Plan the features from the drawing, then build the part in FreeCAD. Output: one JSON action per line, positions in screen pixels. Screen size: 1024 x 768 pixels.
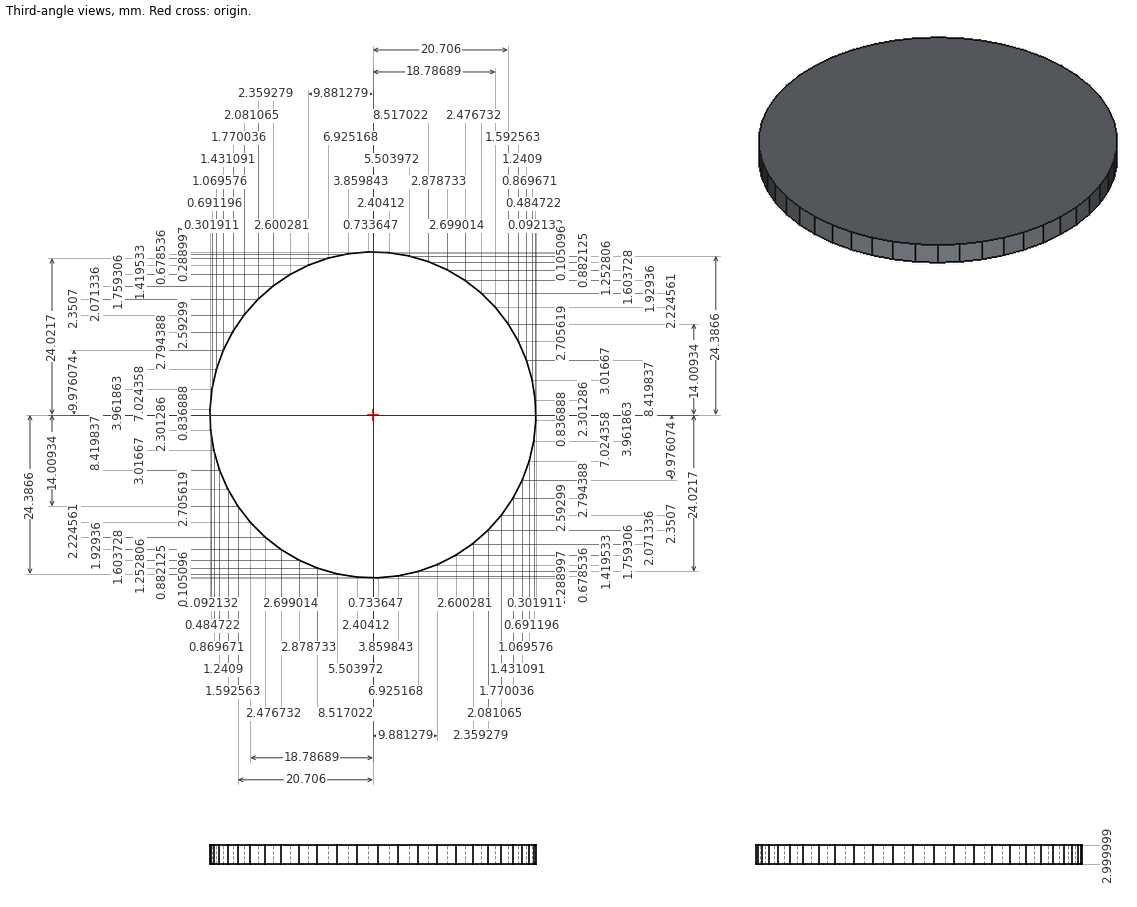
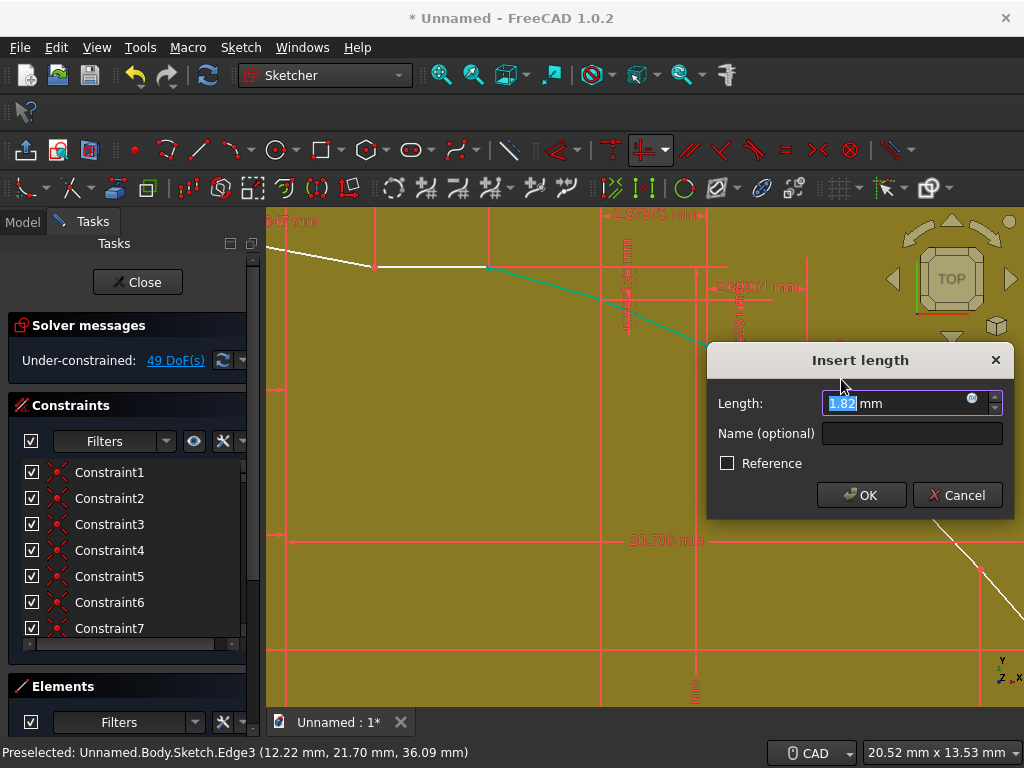
{"action": "type", "text": "1.603728"}
{"action": "key", "text": "Return"}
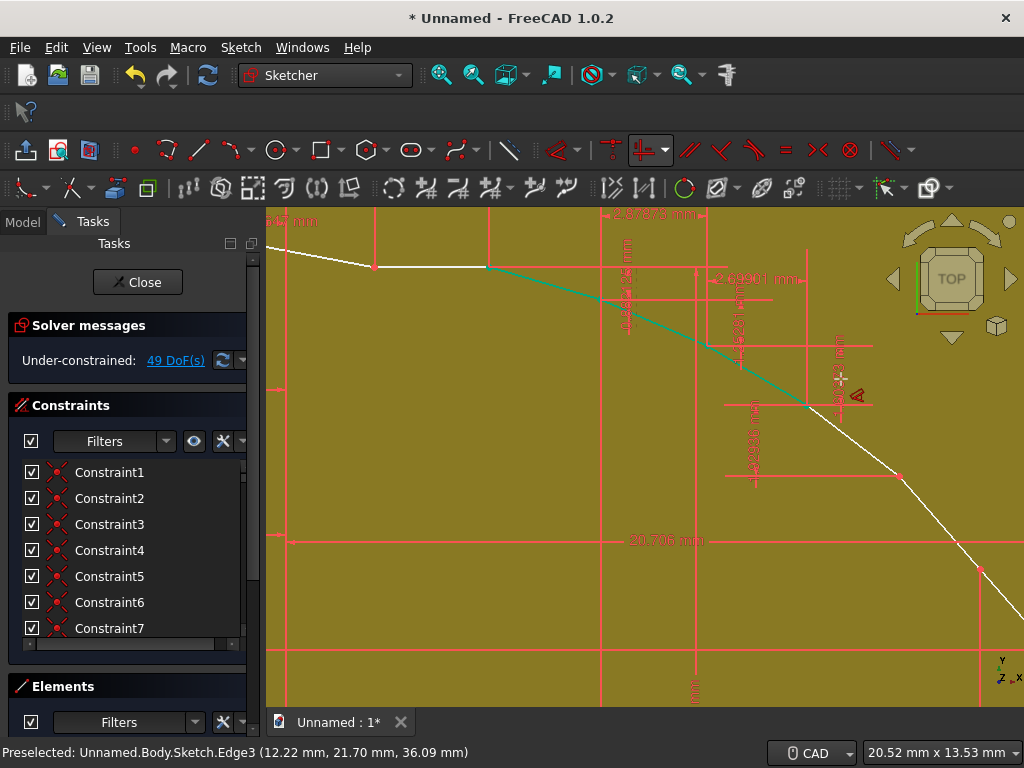
{"action": "left_click", "coordinate": [835, 427]}
{"action": "left_click", "coordinate": [833, 510]}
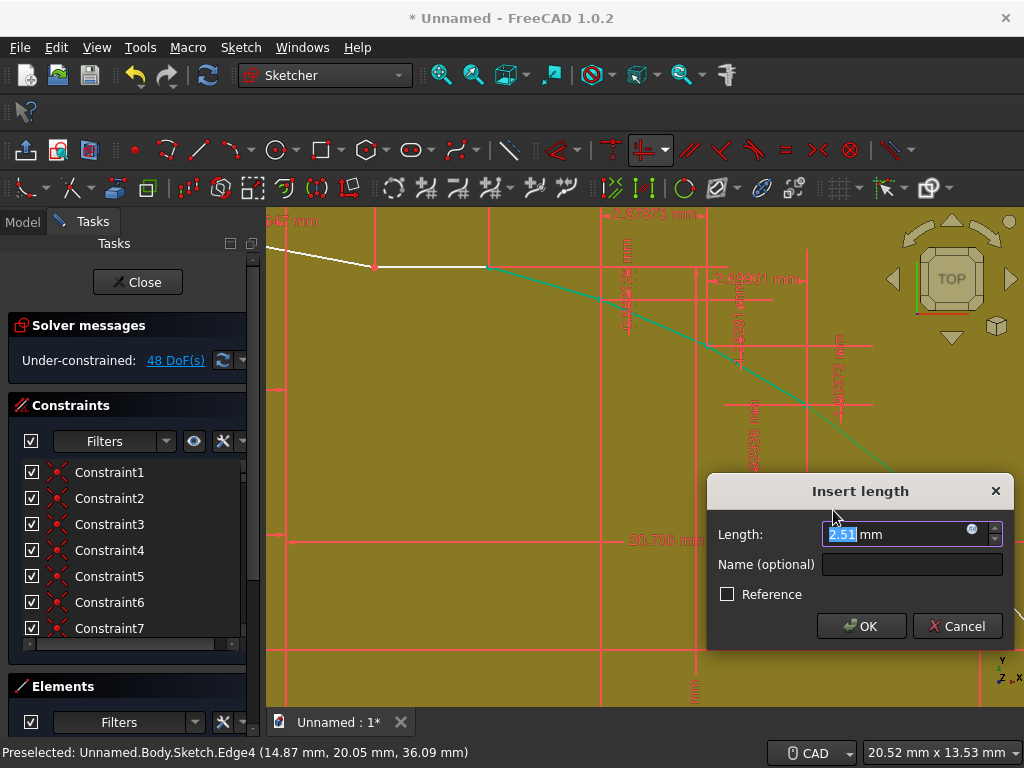
{"action": "type", "text": "2.476732"}
{"action": "key", "text": "Return"}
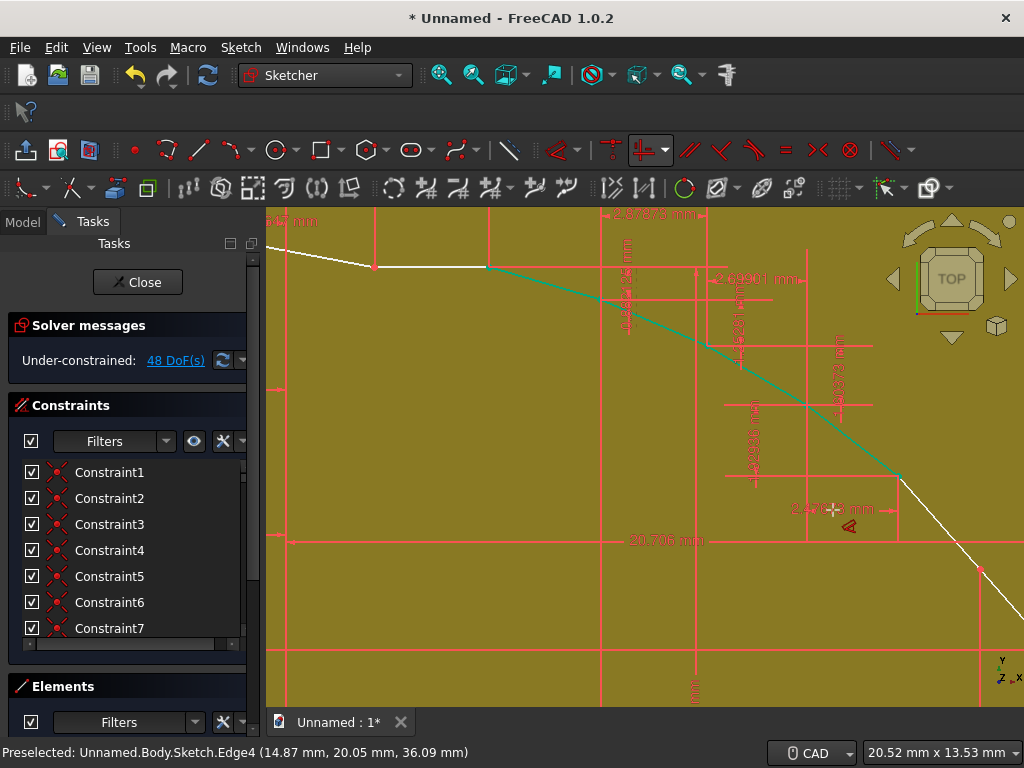
{"action": "scroll", "coordinate": [634, 316], "scroll_direction": "down", "scroll_amount": 9}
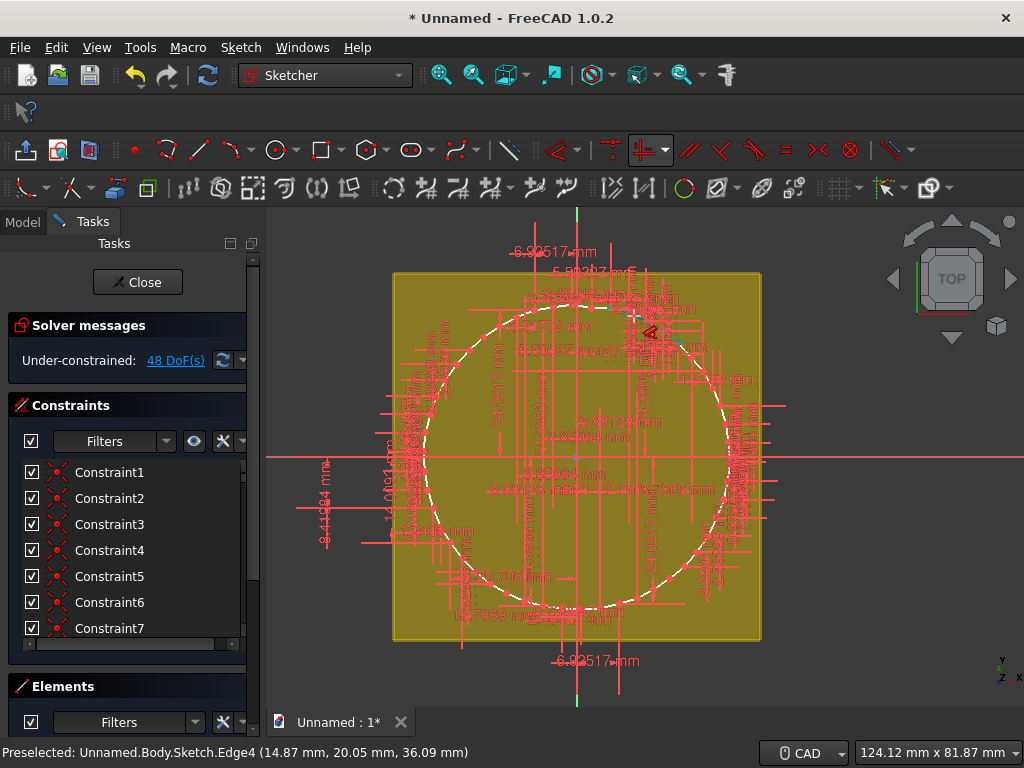
{"action": "scroll", "coordinate": [682, 347], "scroll_direction": "up", "scroll_amount": 6}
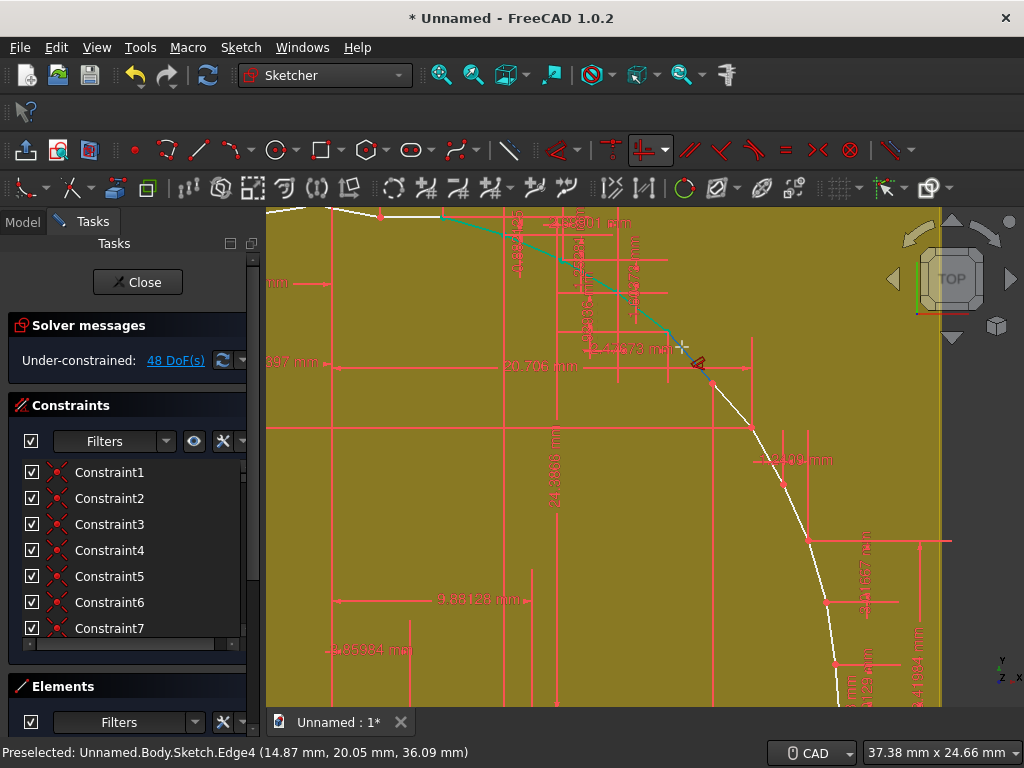
{"action": "left_click", "coordinate": [681, 347]}
{"action": "left_click", "coordinate": [747, 358]}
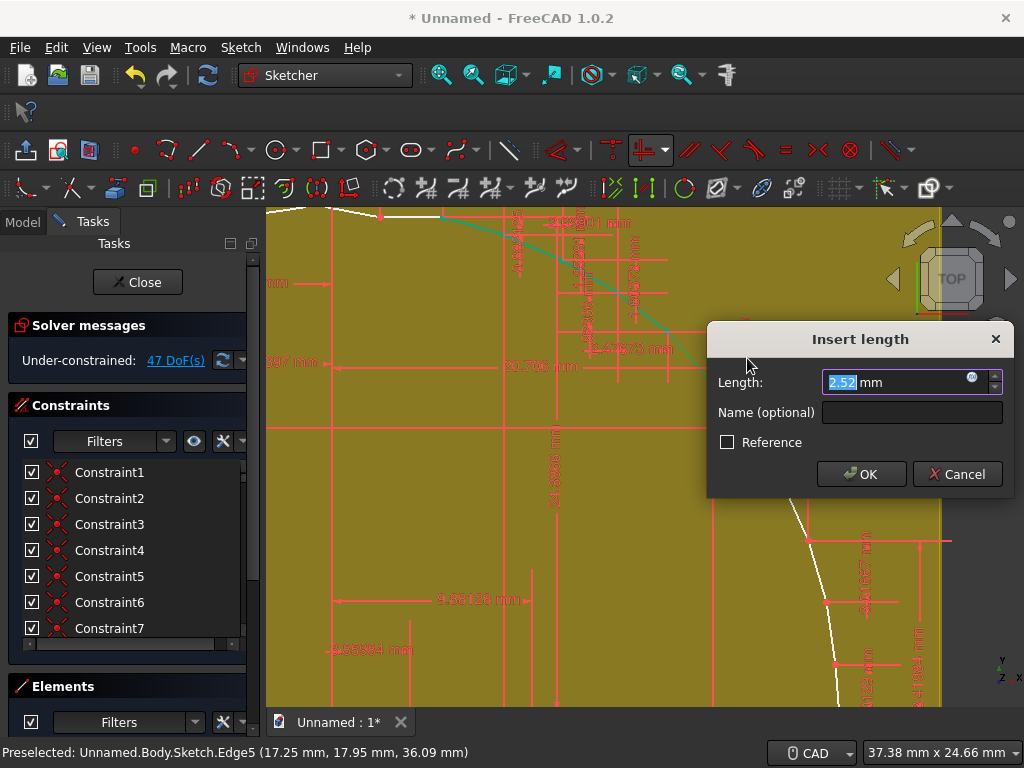
{"action": "type", "text": "2.224561"}
{"action": "key", "text": "Return"}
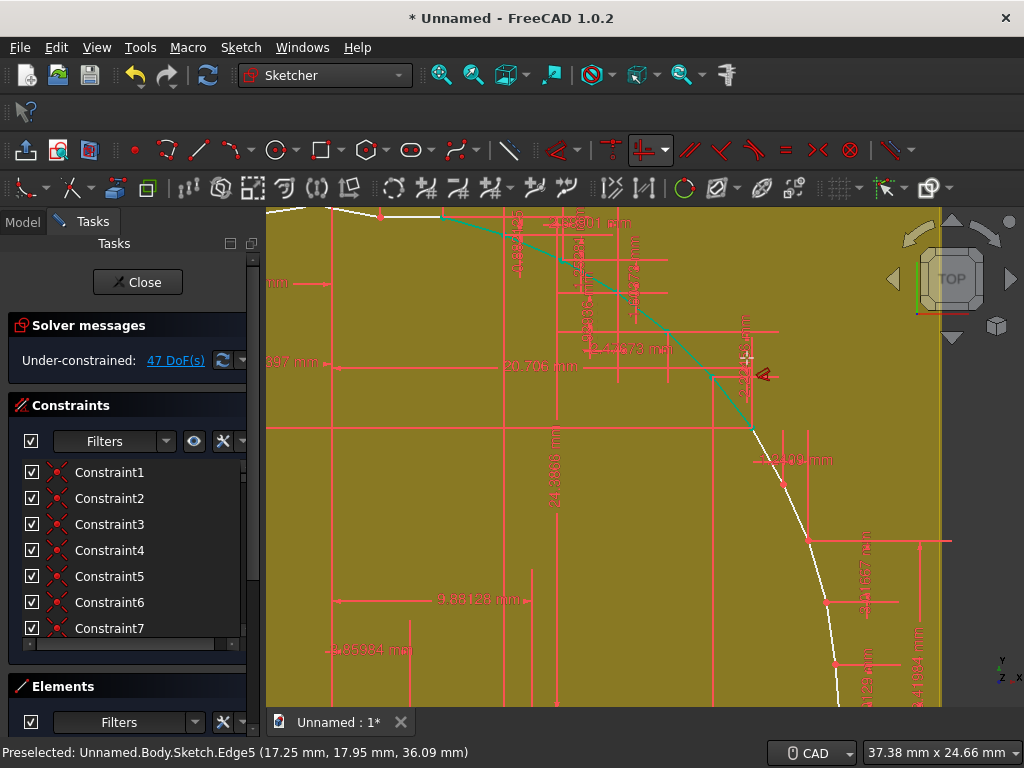
{"action": "scroll", "coordinate": [761, 445], "scroll_direction": "up", "scroll_amount": 2}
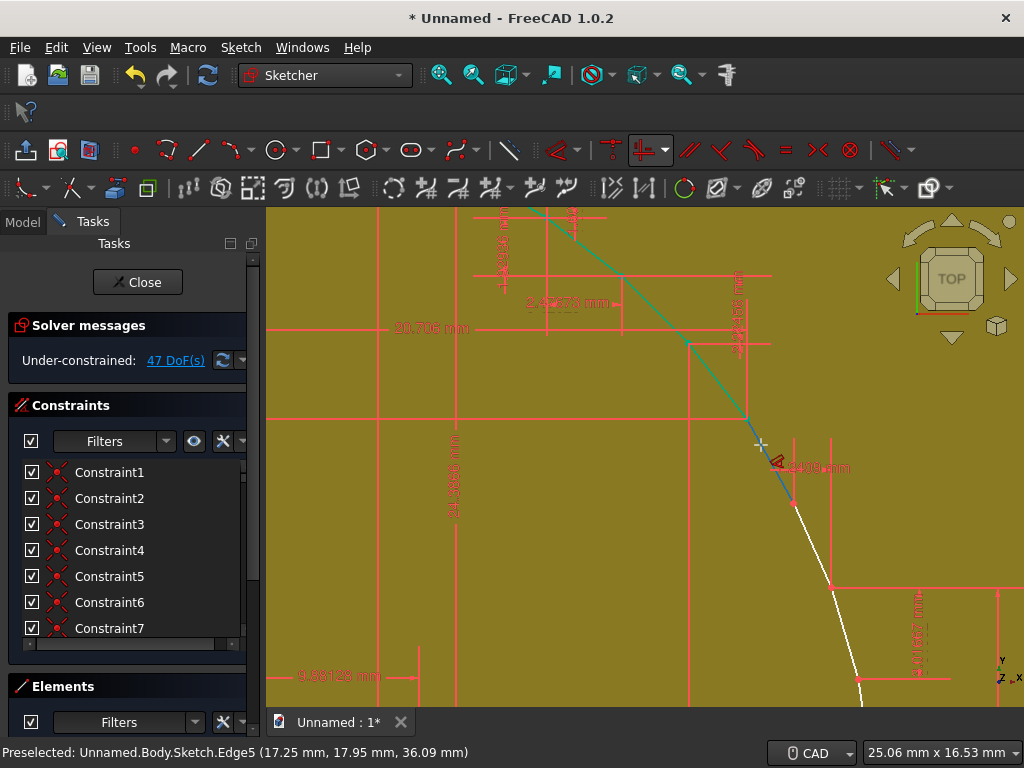
{"action": "left_click", "coordinate": [761, 444]}
{"action": "left_click", "coordinate": [770, 385]}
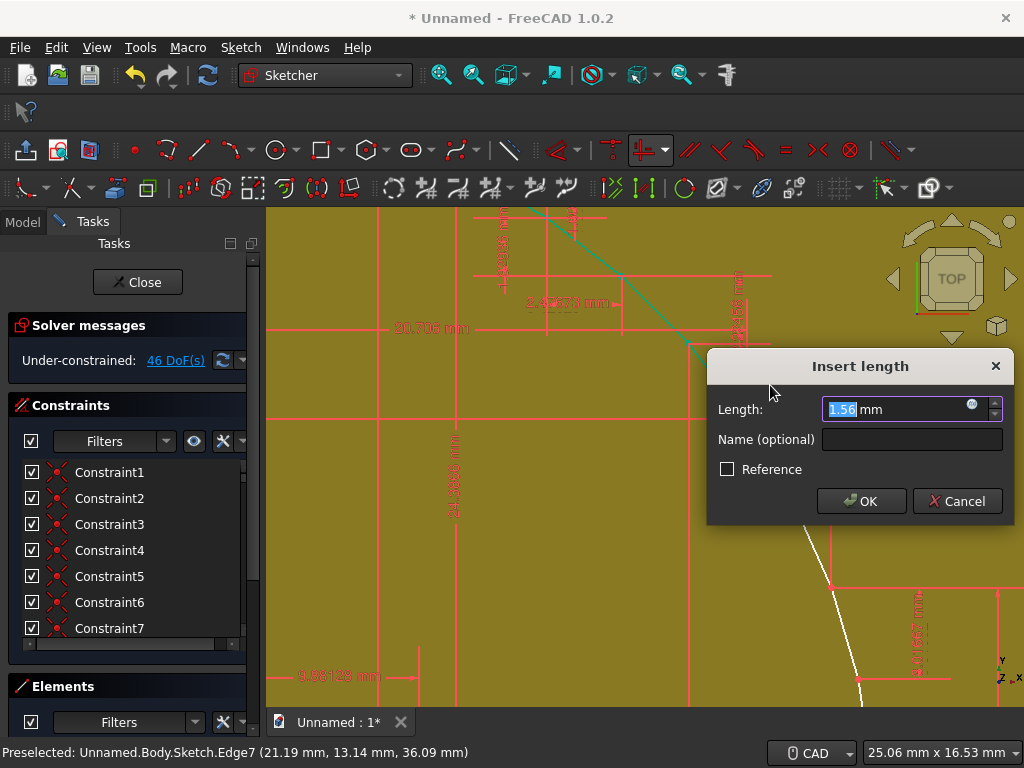
{"action": "type", "text": "1.592563"}
{"action": "key", "text": "Return"}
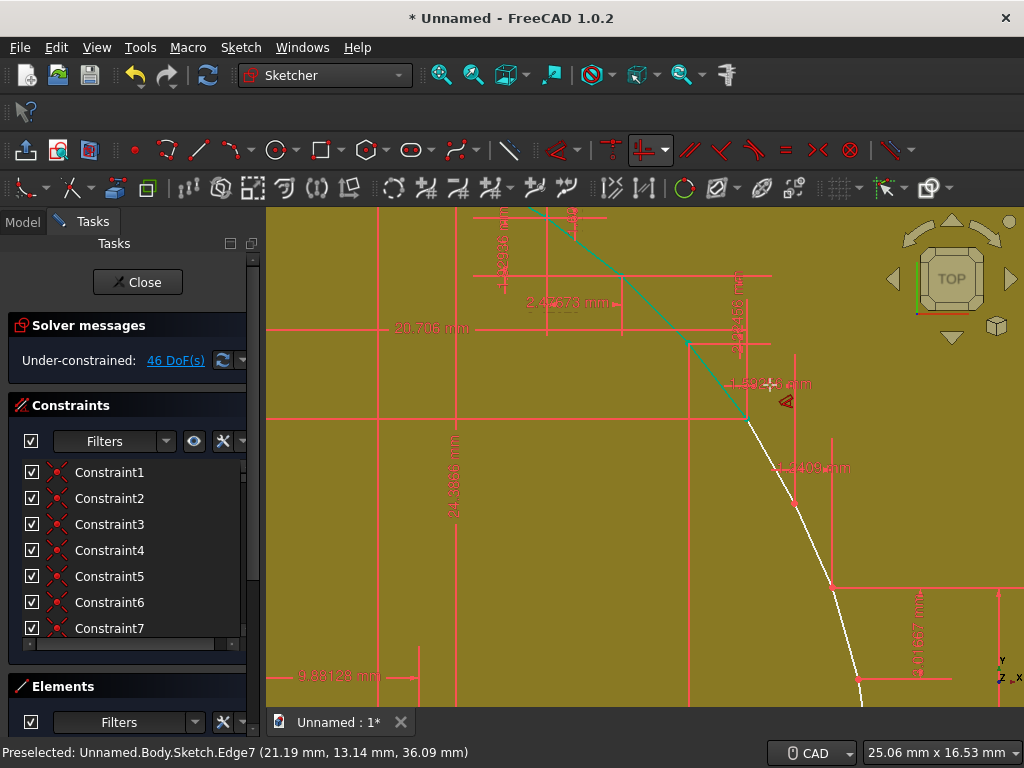
{"action": "left_click", "coordinate": [761, 444]}
{"action": "left_click", "coordinate": [829, 442]}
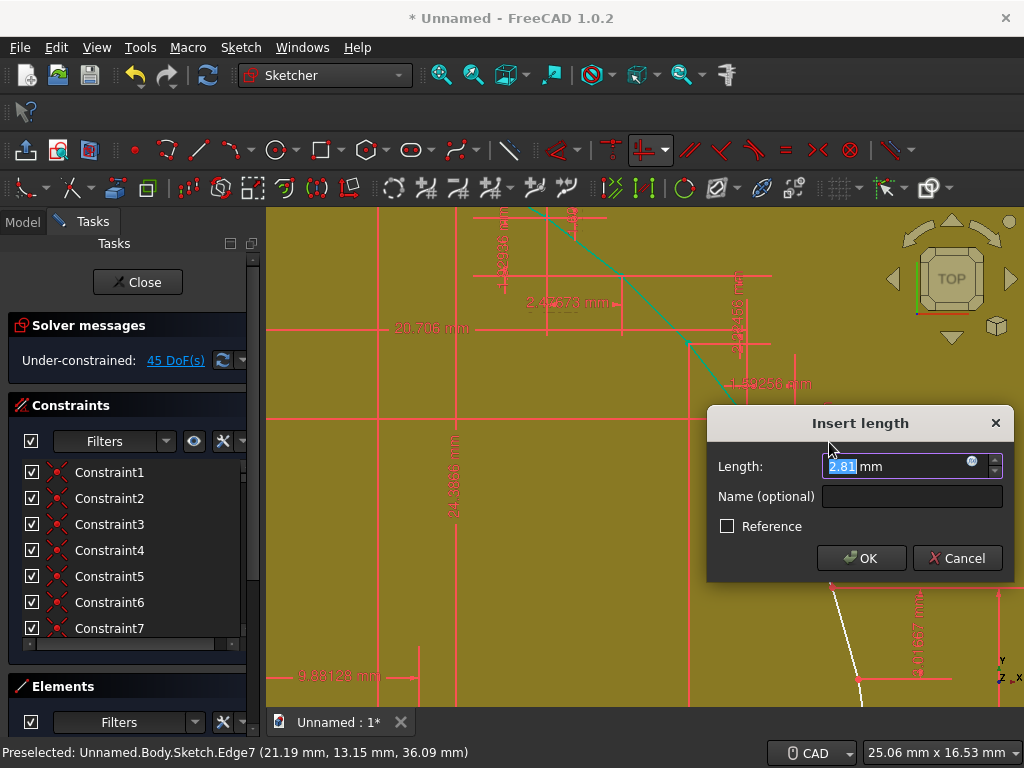
{"action": "type", "text": "2.705619"}
{"action": "key", "text": "Return"}